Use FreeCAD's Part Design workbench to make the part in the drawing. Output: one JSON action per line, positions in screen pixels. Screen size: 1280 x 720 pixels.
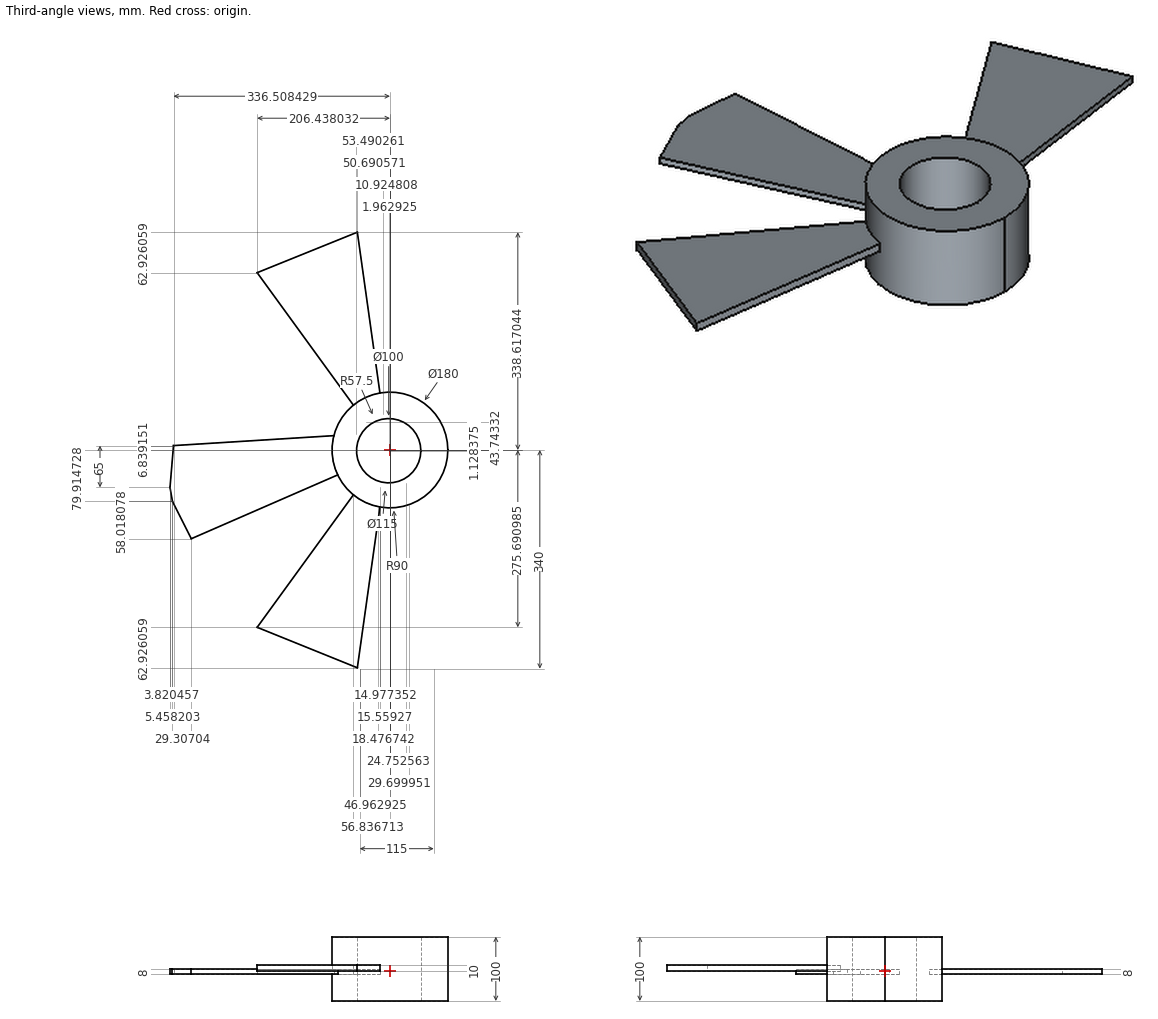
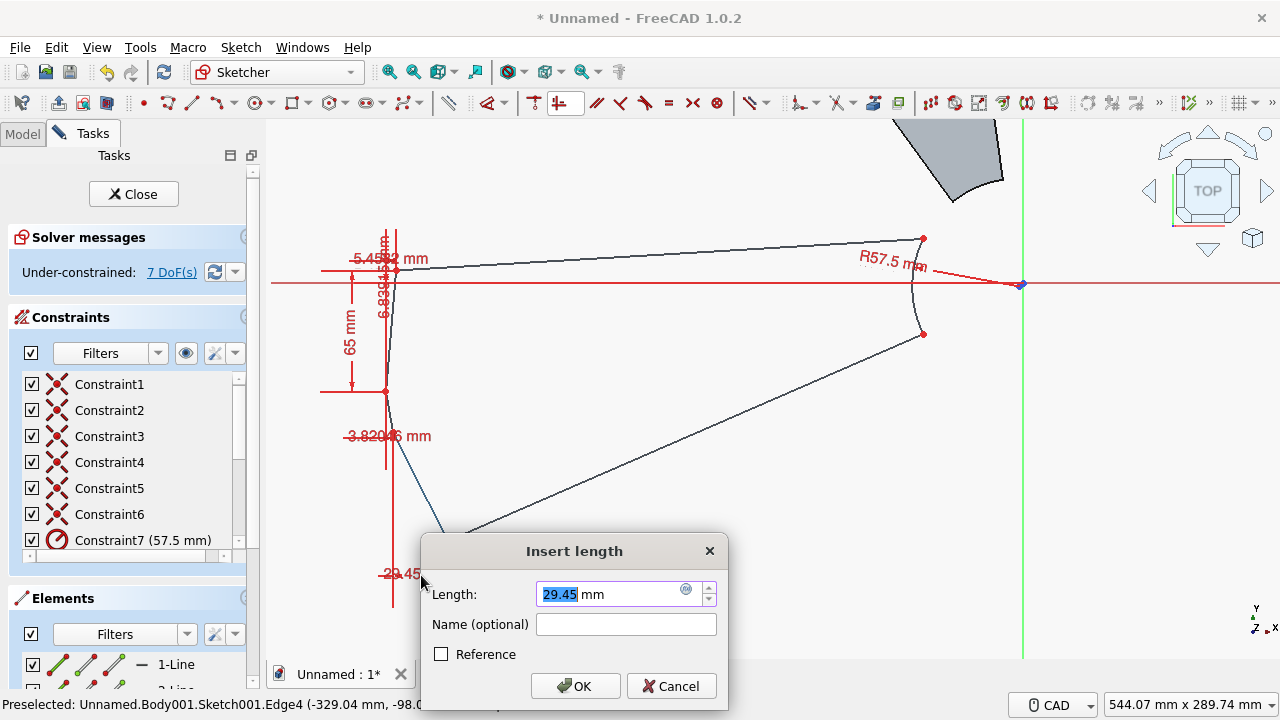
{"action": "type", "text": "29.30704"}
{"action": "key", "text": "Return"}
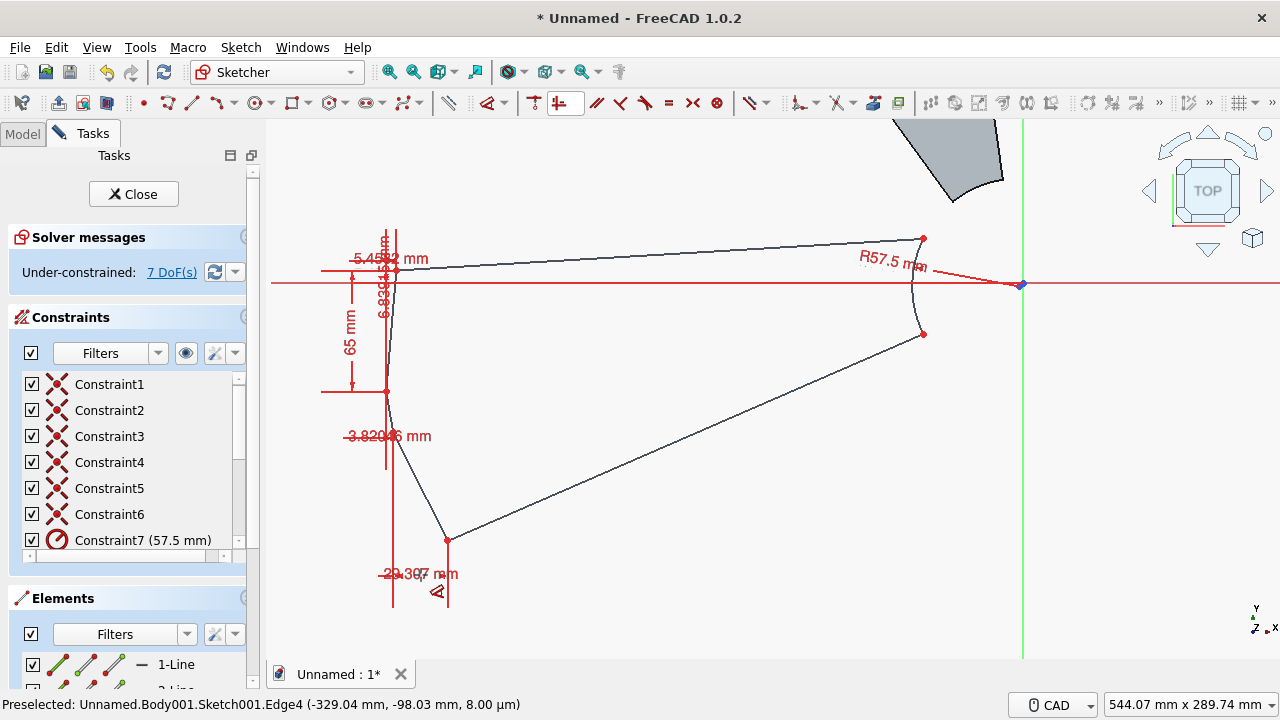
{"action": "scroll", "coordinate": [1019, 286], "scroll_direction": "up", "scroll_amount": 12}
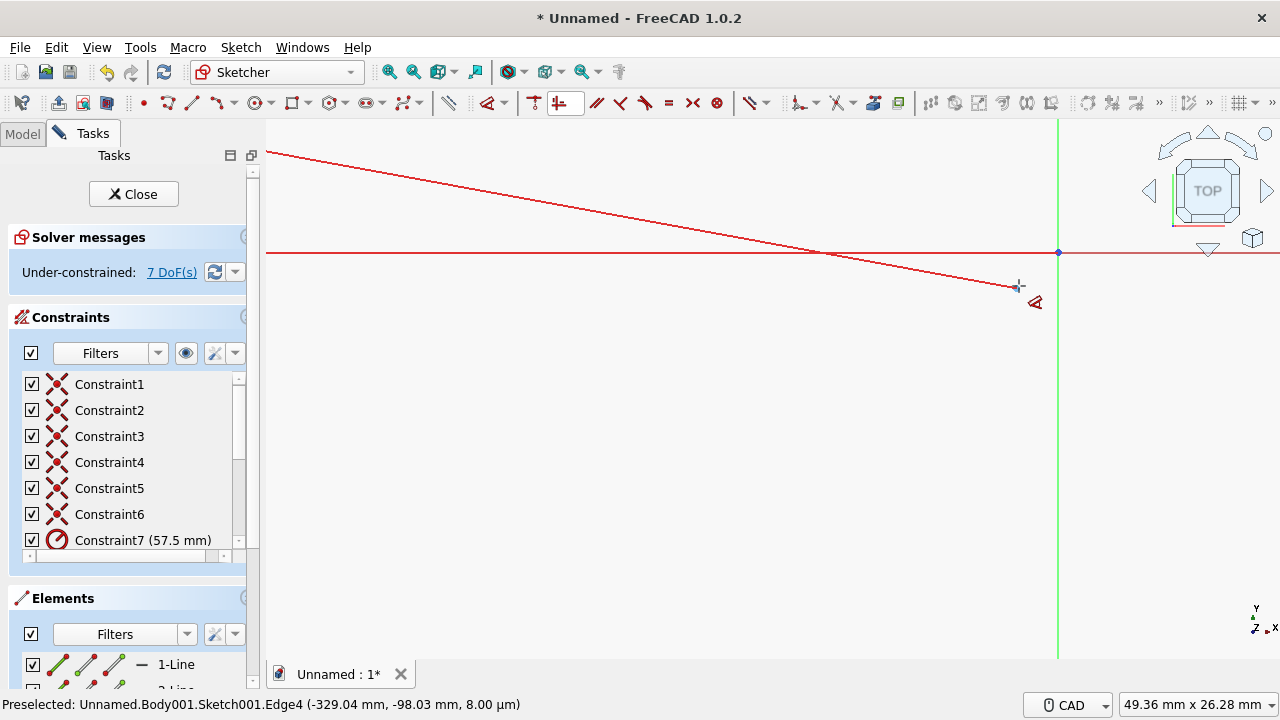
{"action": "left_click", "coordinate": [1016, 288]}
{"action": "left_click", "coordinate": [1037, 219]}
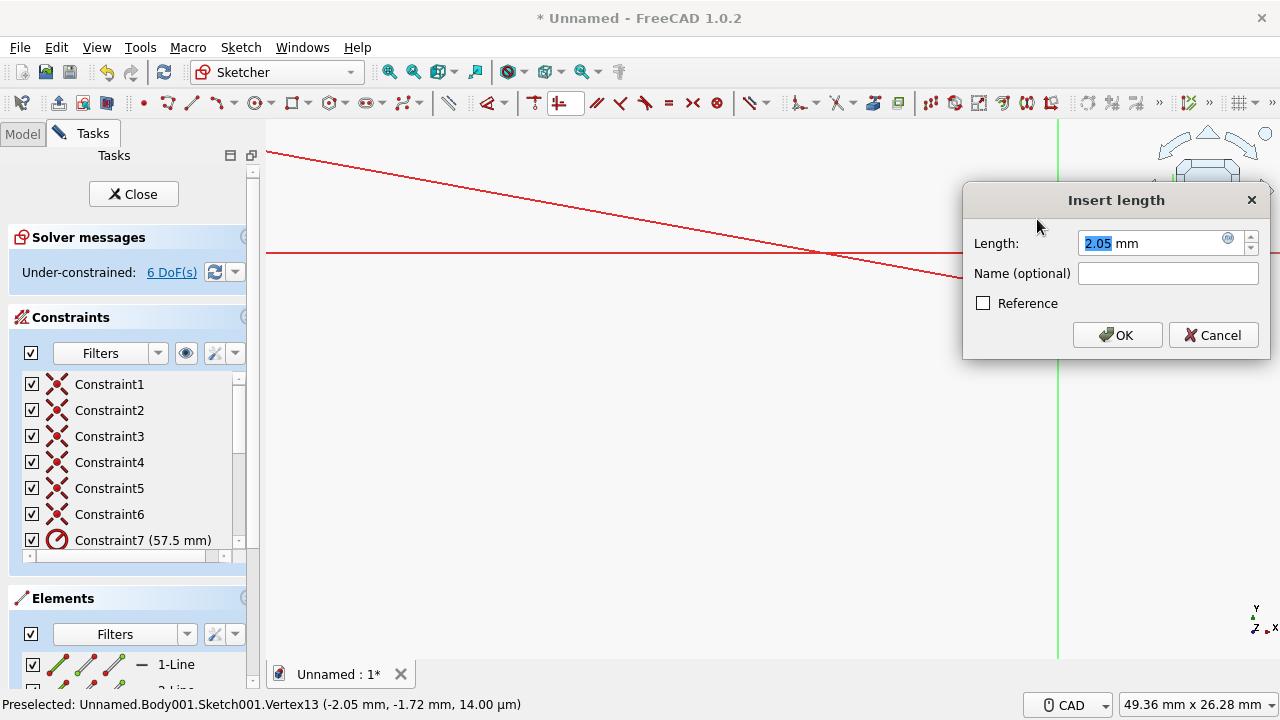
{"action": "type", "text": "1.962925"}
{"action": "key", "text": "Return"}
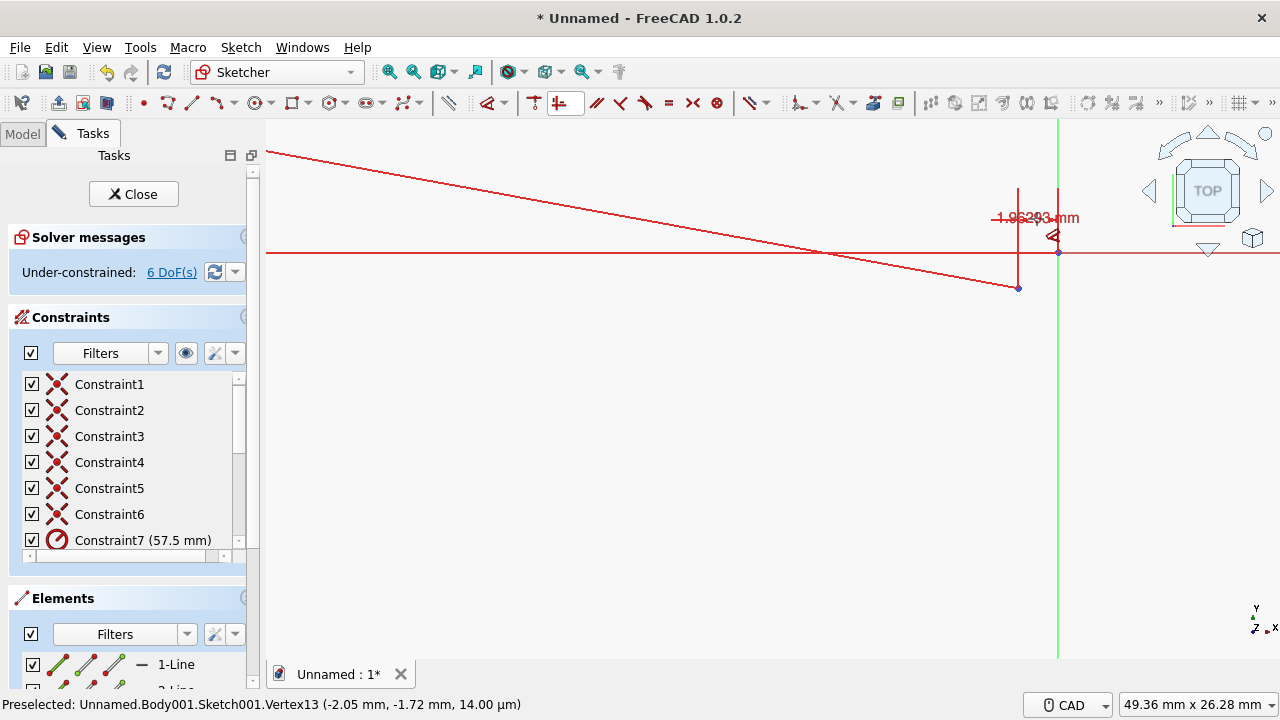
{"action": "scroll", "coordinate": [1018, 288], "scroll_direction": "up", "scroll_amount": 3}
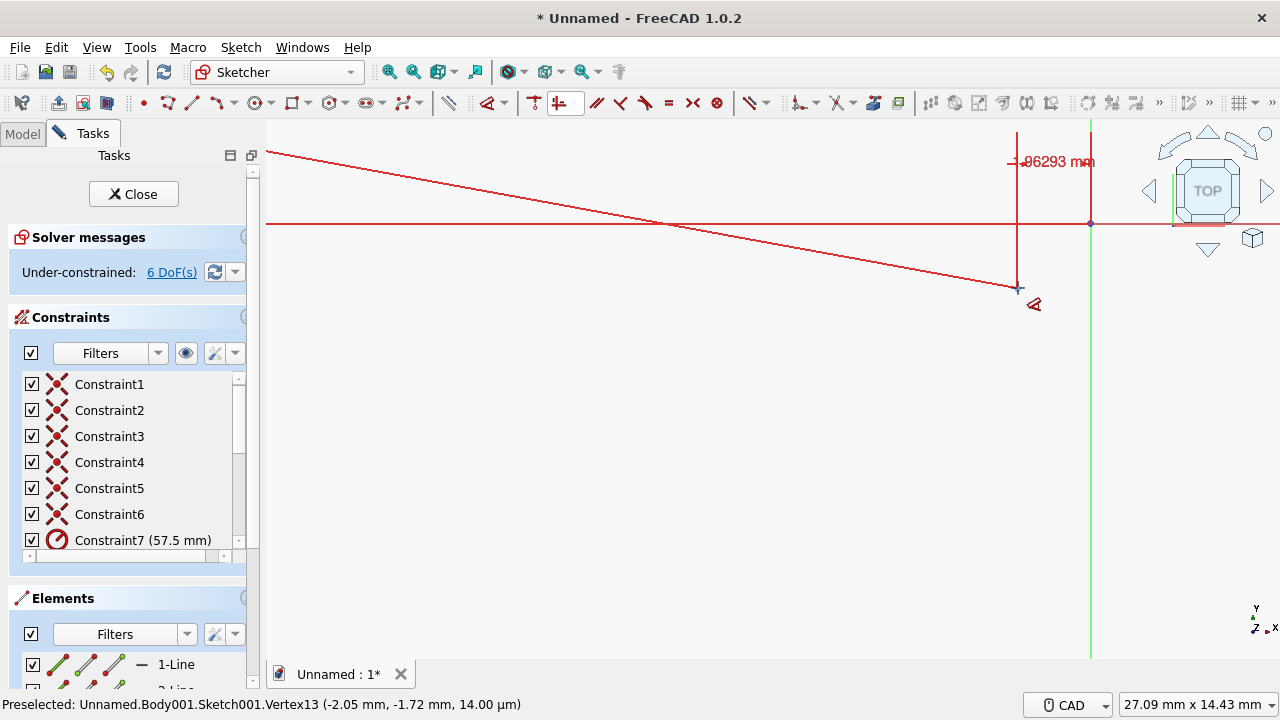
{"action": "left_click", "coordinate": [1017, 288]}
{"action": "left_click", "coordinate": [983, 256]}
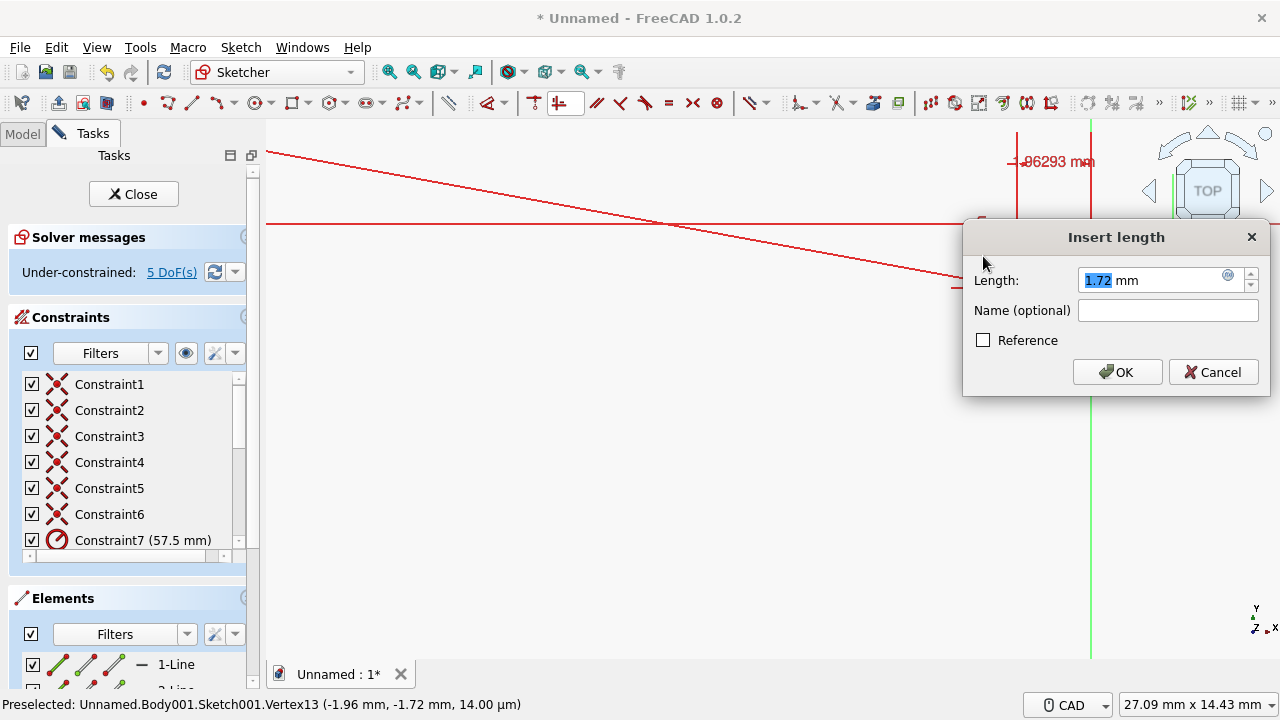
{"action": "type", "text": "1.128375"}
{"action": "key", "text": "Return"}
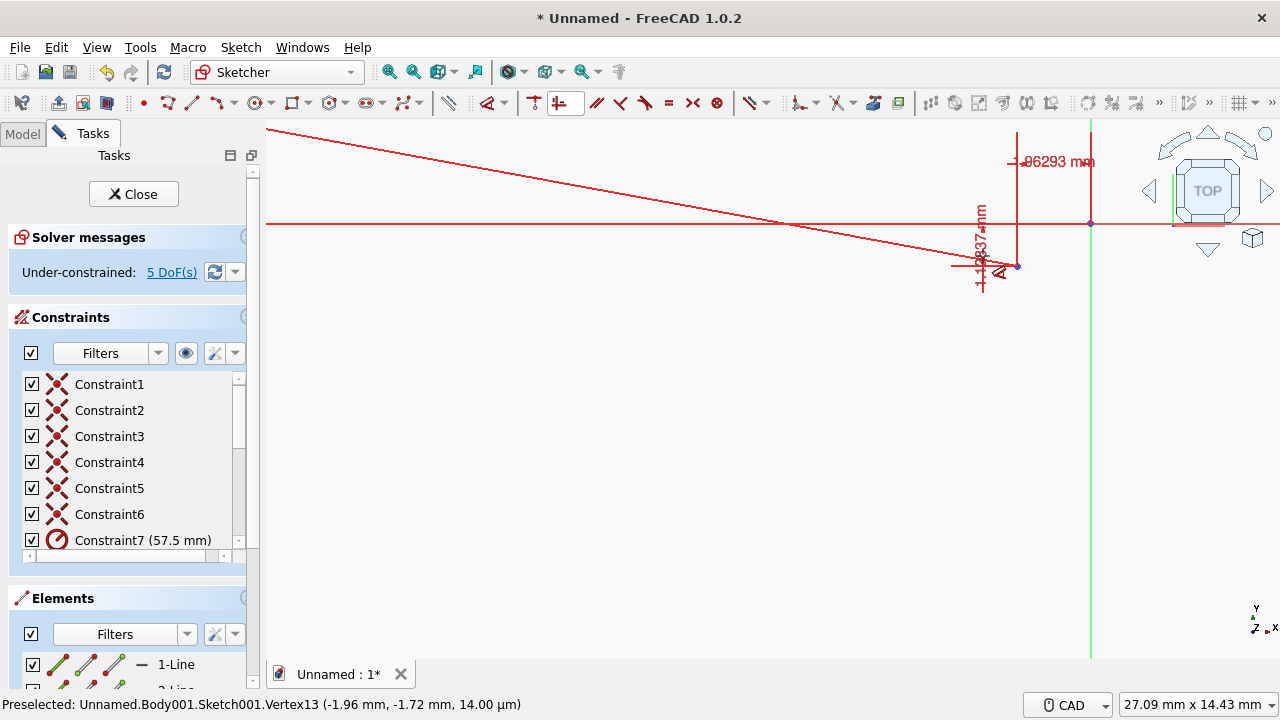
{"action": "scroll", "coordinate": [1020, 286], "scroll_direction": "down", "scroll_amount": 15}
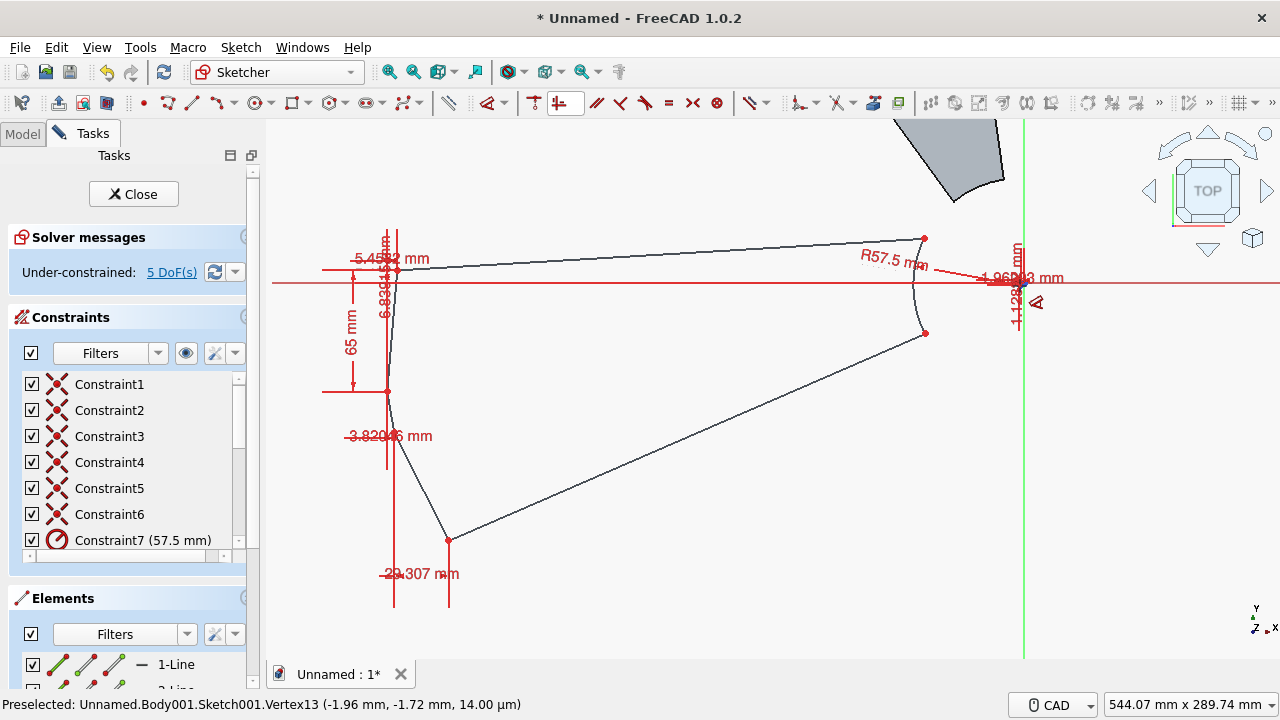
{"action": "left_click", "coordinate": [924, 239]}
{"action": "left_click", "coordinate": [974, 205]}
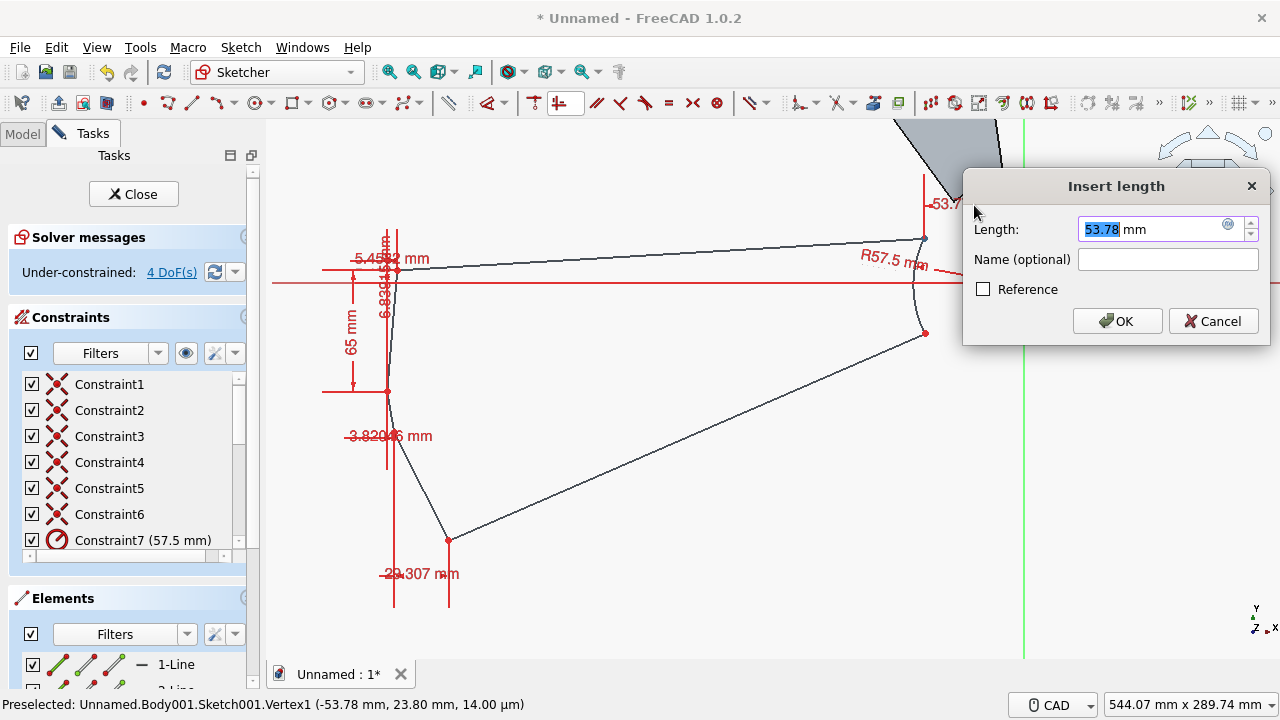
{"action": "type", "text": "53.490261"}
{"action": "key", "text": "Return"}